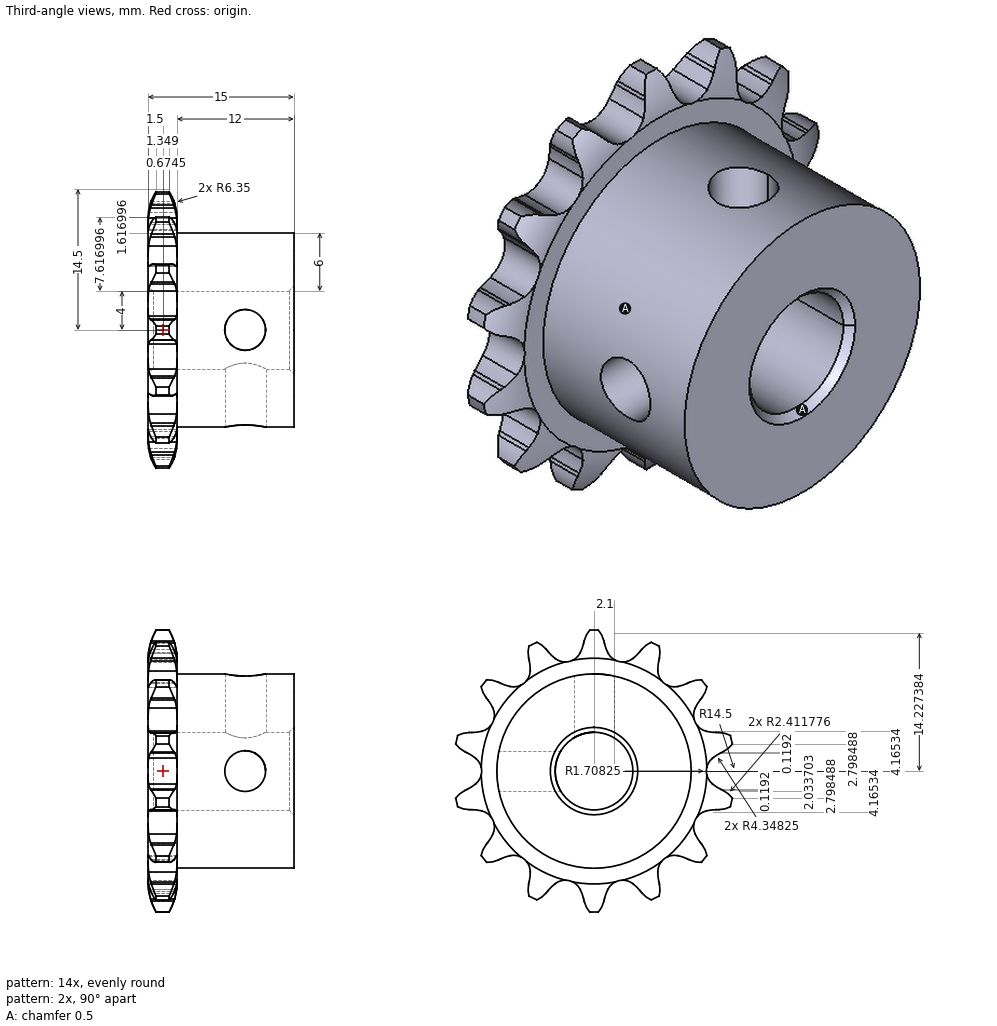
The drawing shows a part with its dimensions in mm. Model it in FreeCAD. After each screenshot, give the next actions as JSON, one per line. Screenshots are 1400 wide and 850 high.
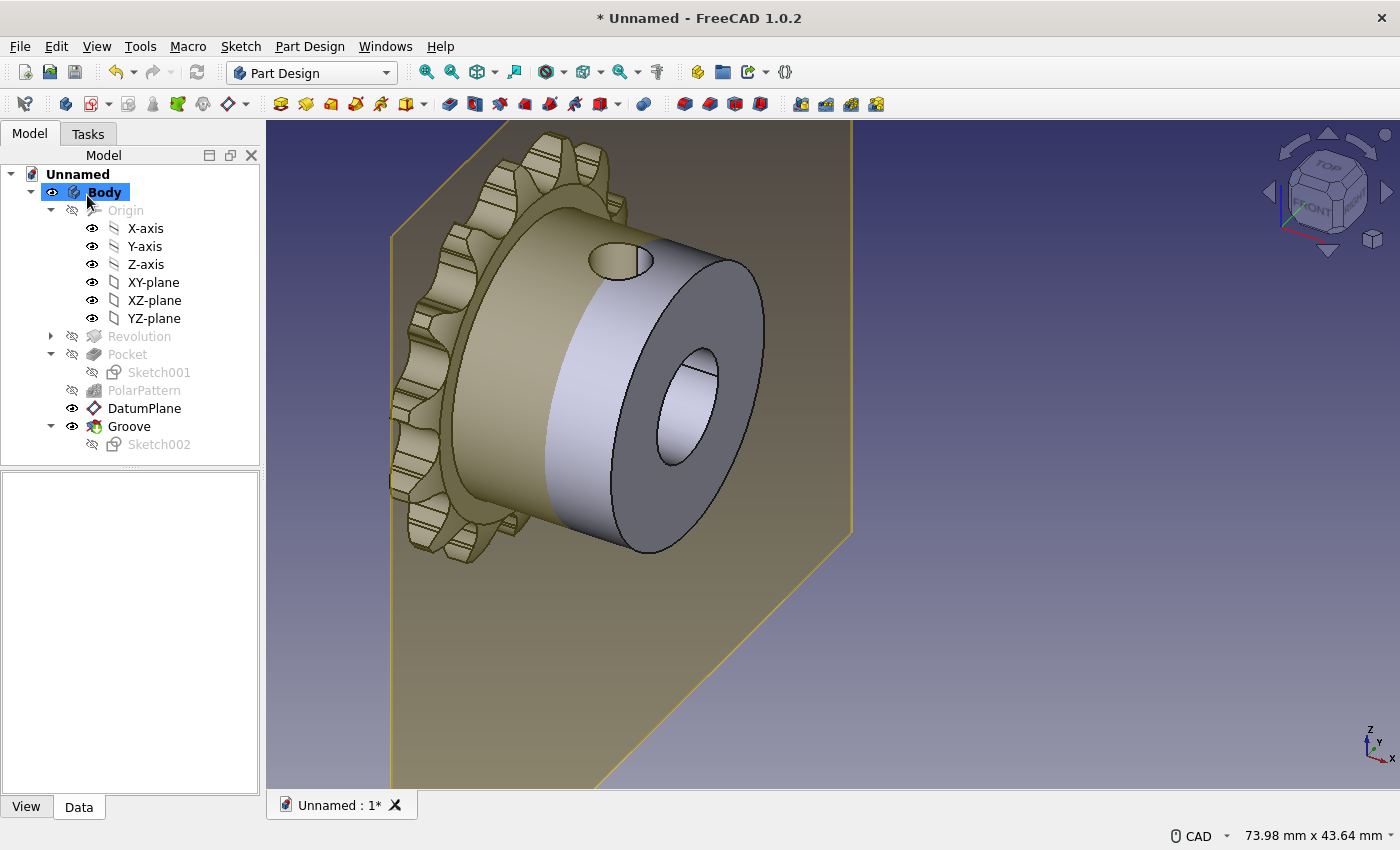
{"action": "left_click", "coordinate": [117, 408]}
{"action": "key", "text": "space"}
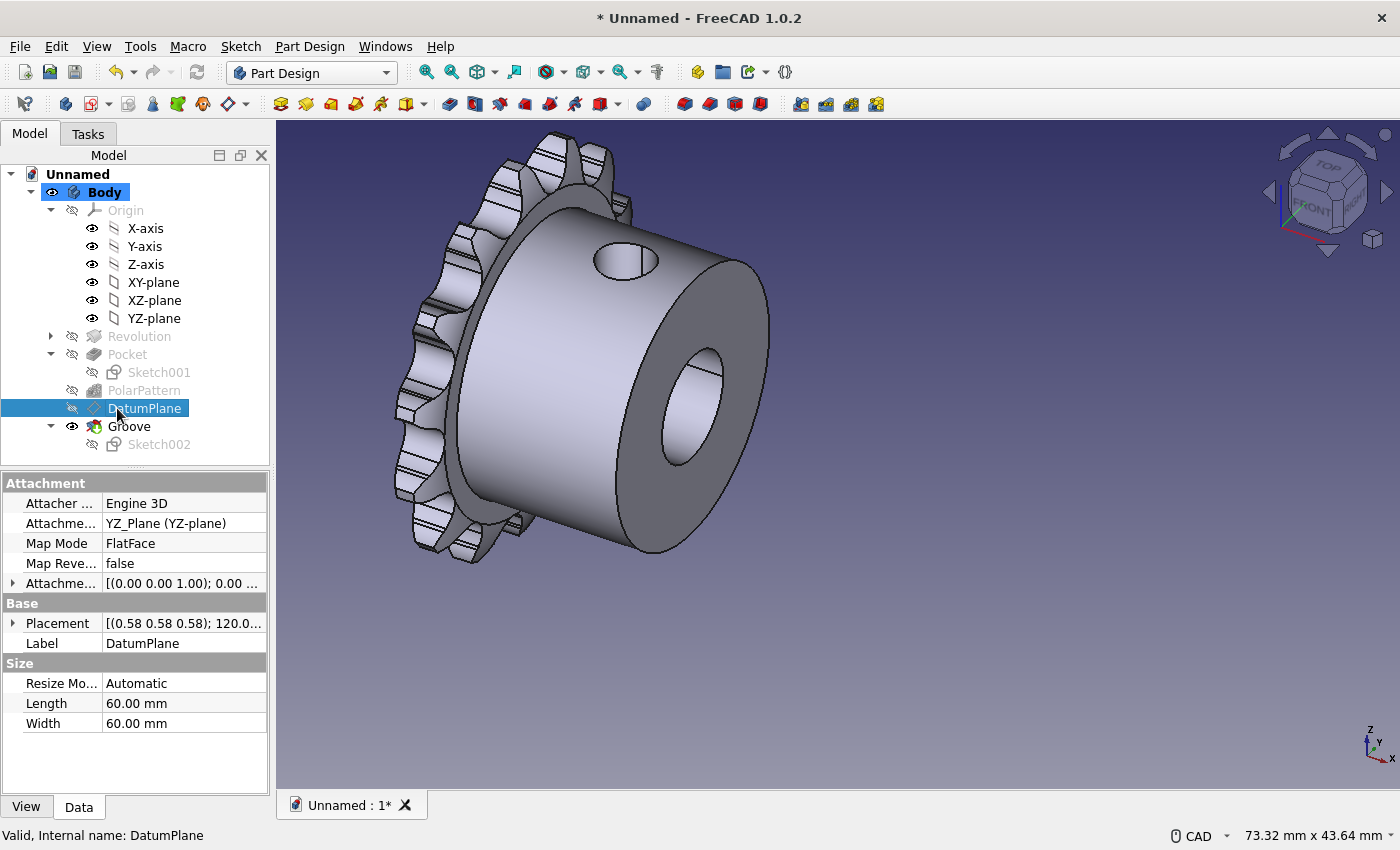
{"action": "left_click", "coordinate": [427, 72]}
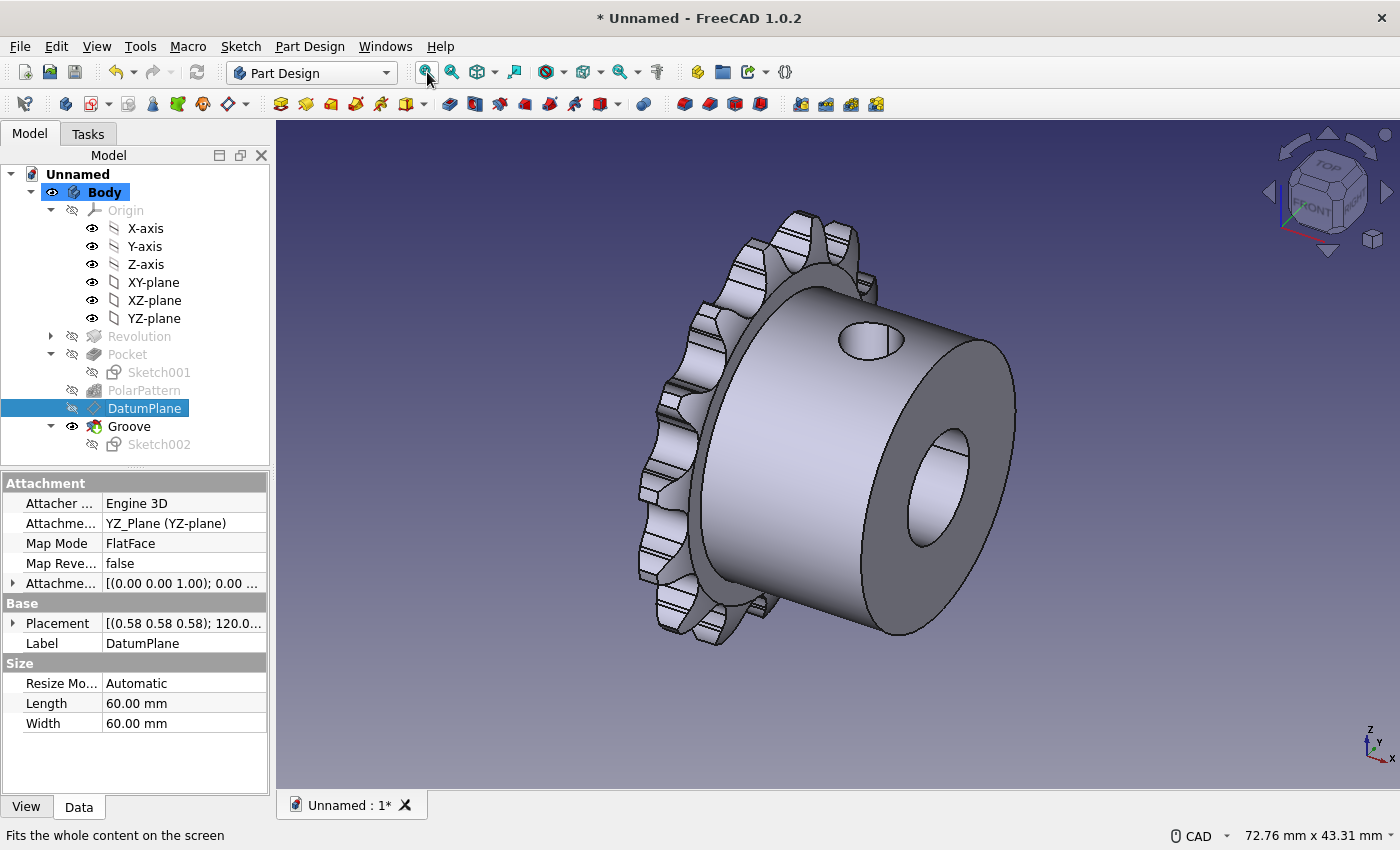
{"action": "left_click", "coordinate": [117, 426]}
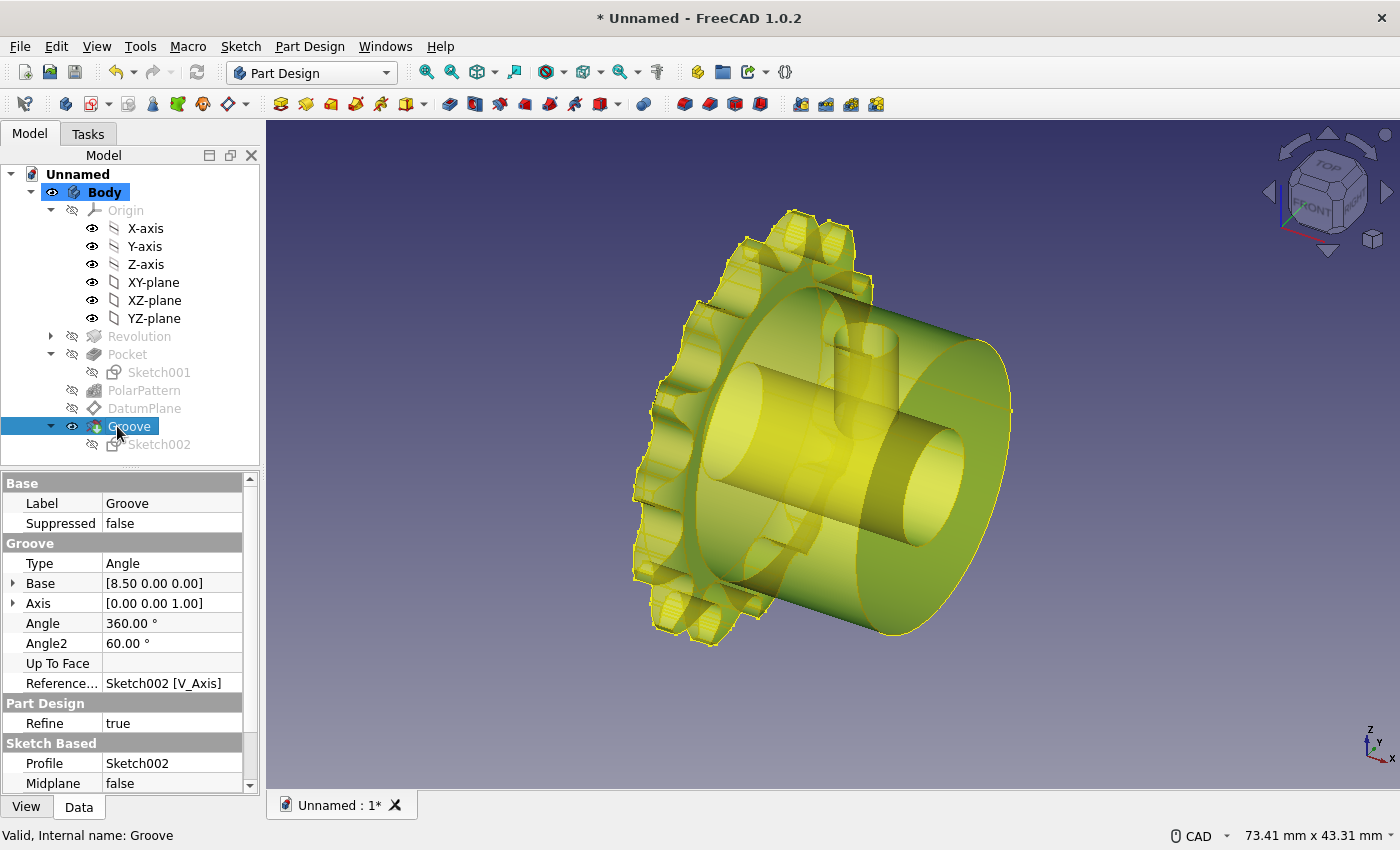
{"action": "left_click", "coordinate": [851, 104]}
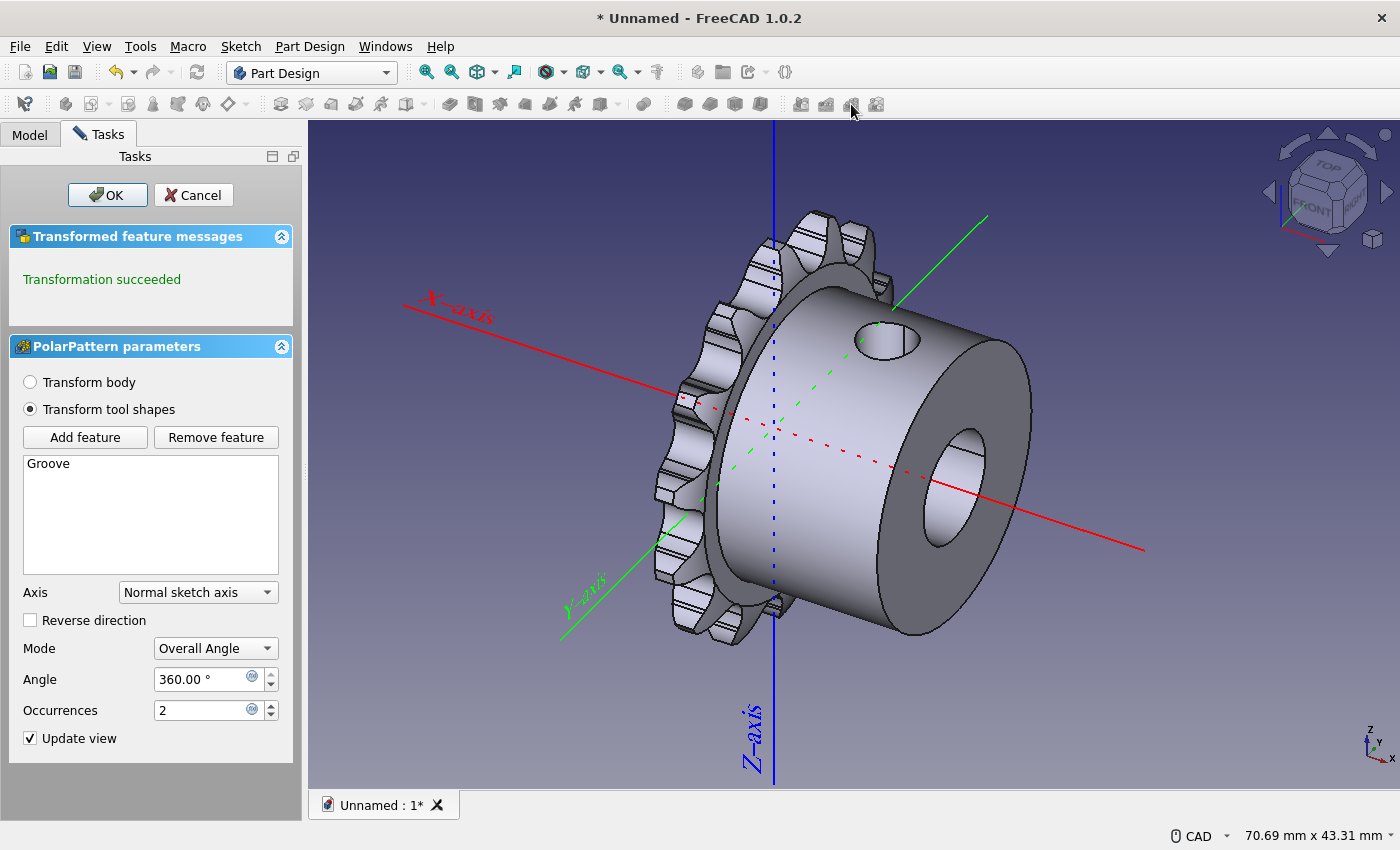
{"action": "left_click", "coordinate": [199, 592]}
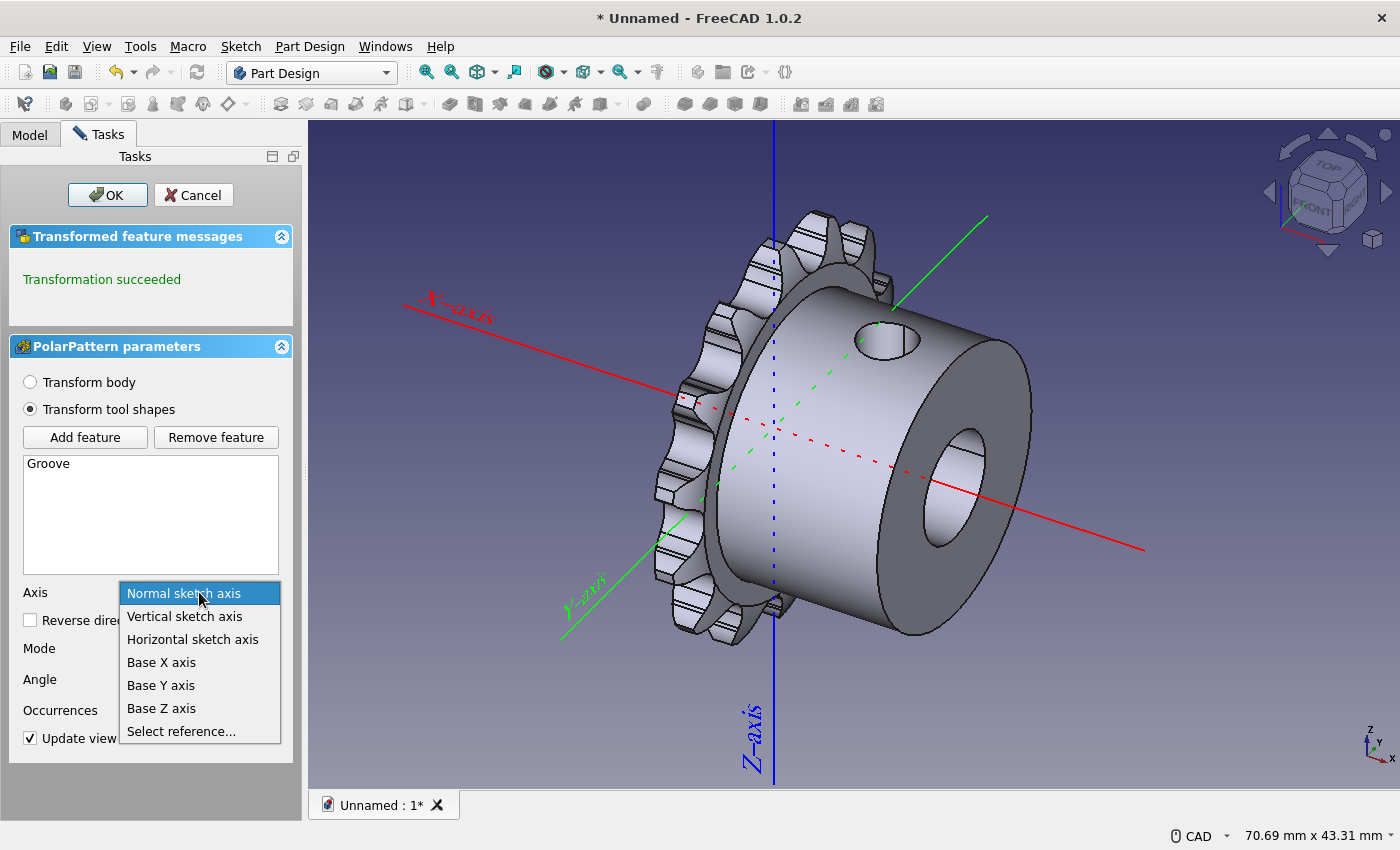
{"action": "left_click", "coordinate": [198, 662]}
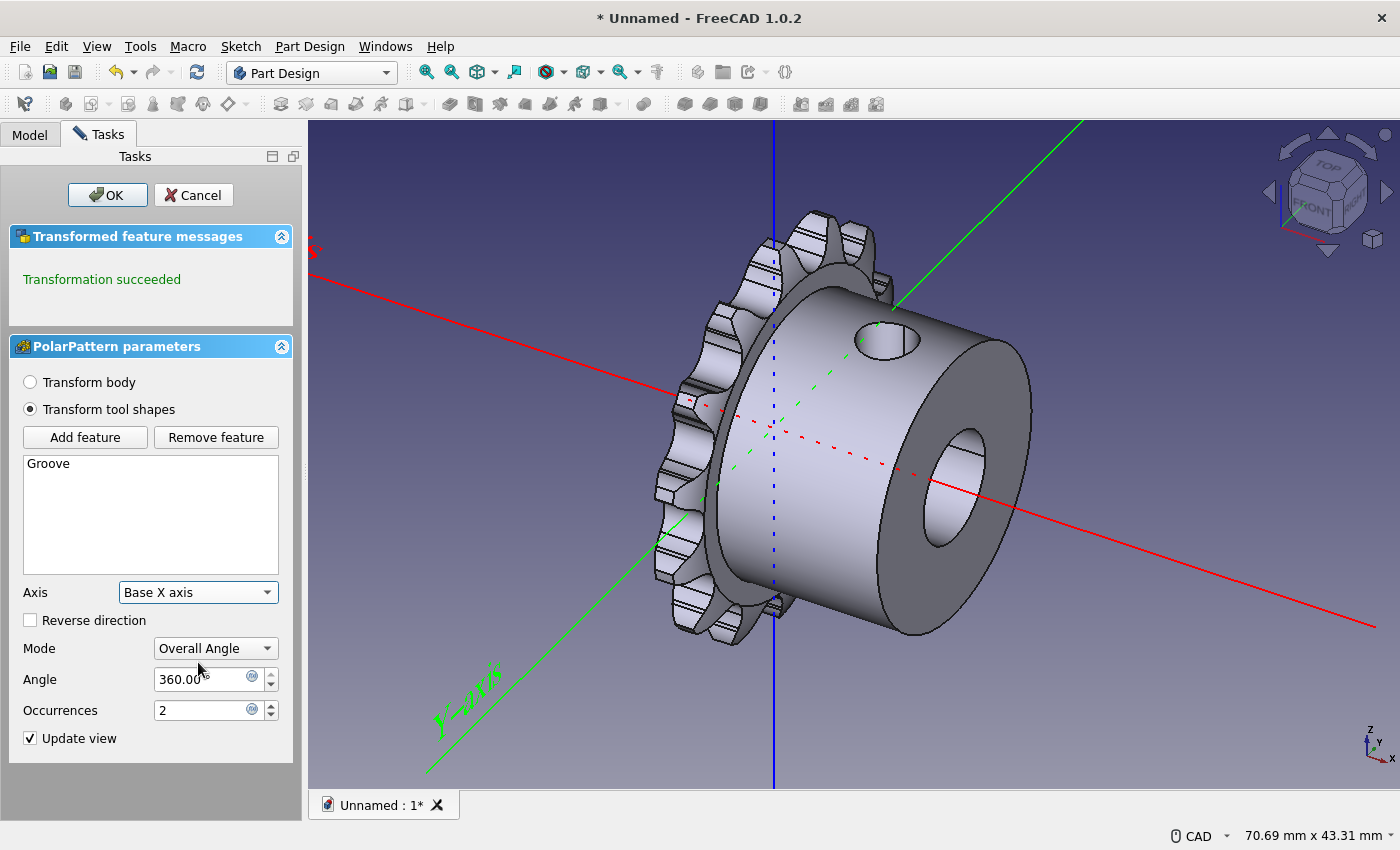
{"action": "left_click", "coordinate": [216, 648]}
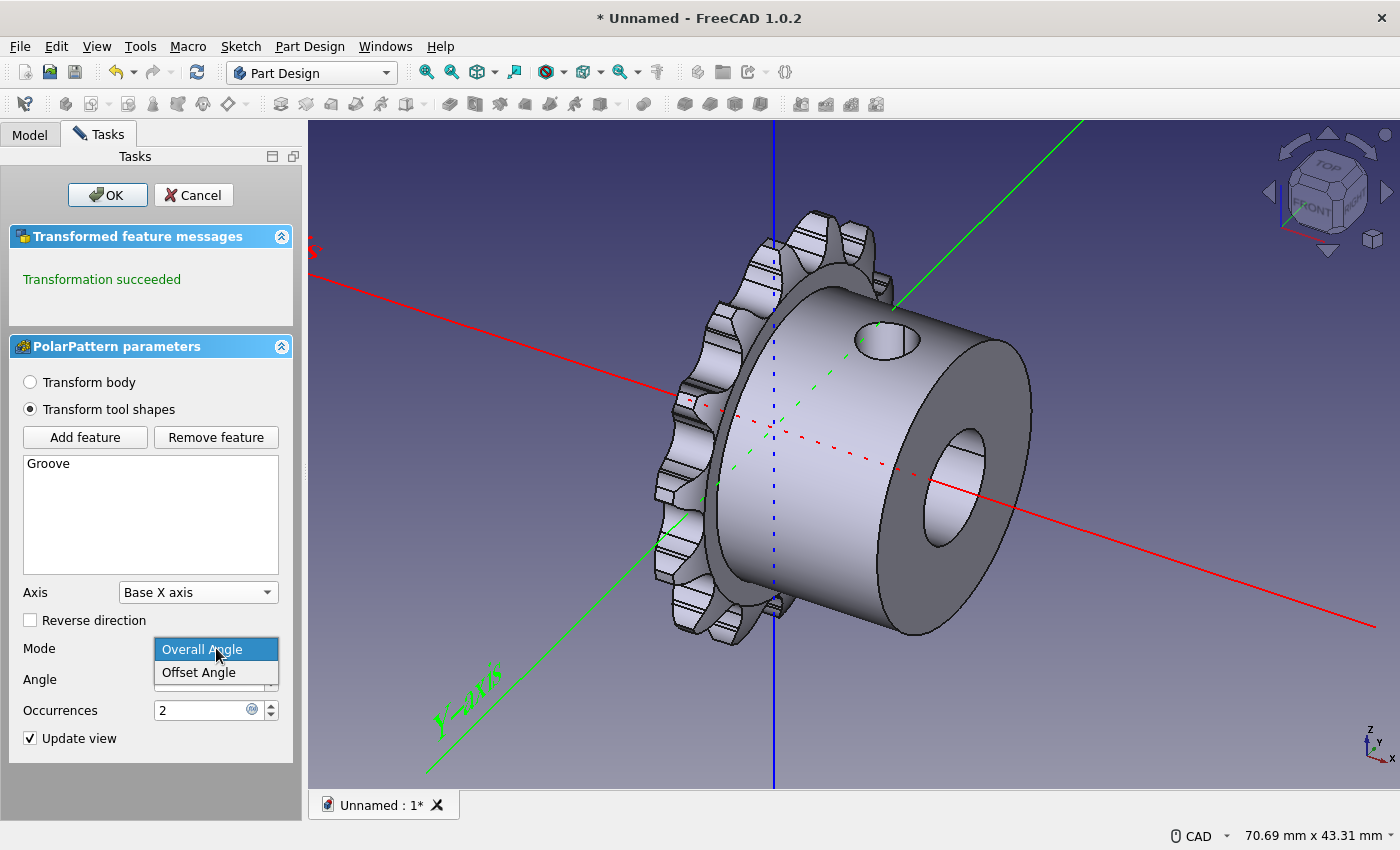
{"action": "left_click", "coordinate": [214, 672]}